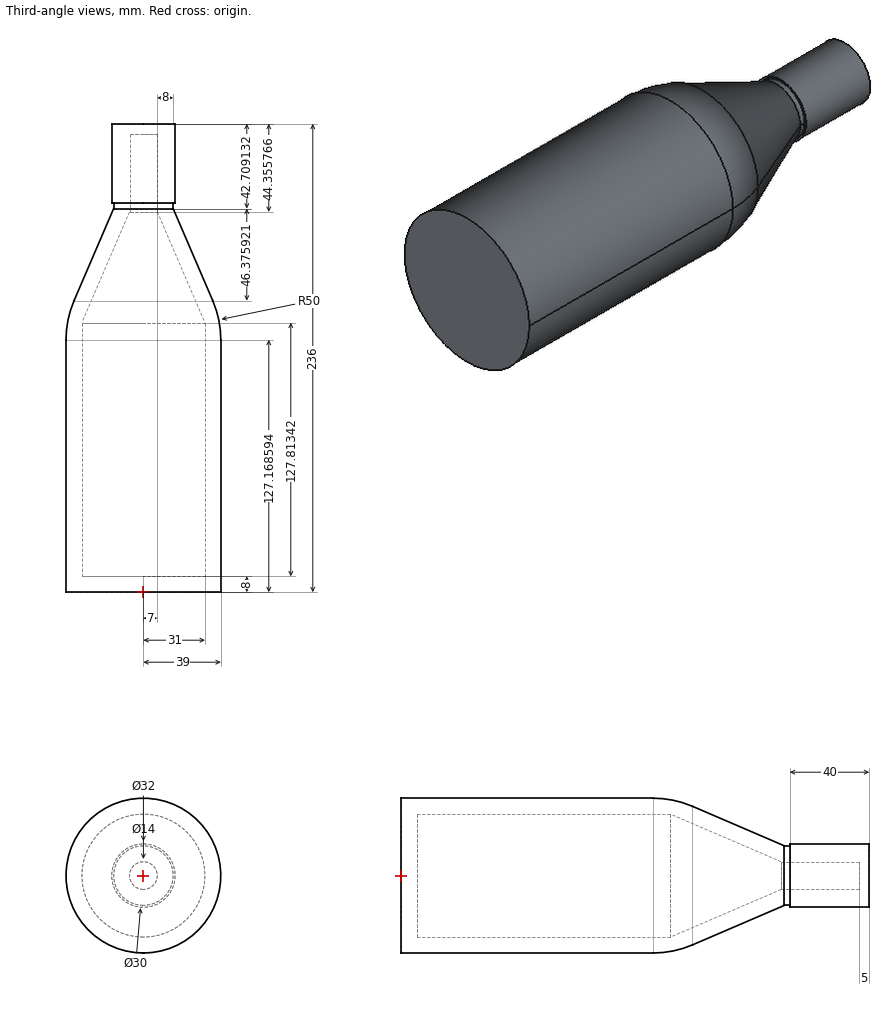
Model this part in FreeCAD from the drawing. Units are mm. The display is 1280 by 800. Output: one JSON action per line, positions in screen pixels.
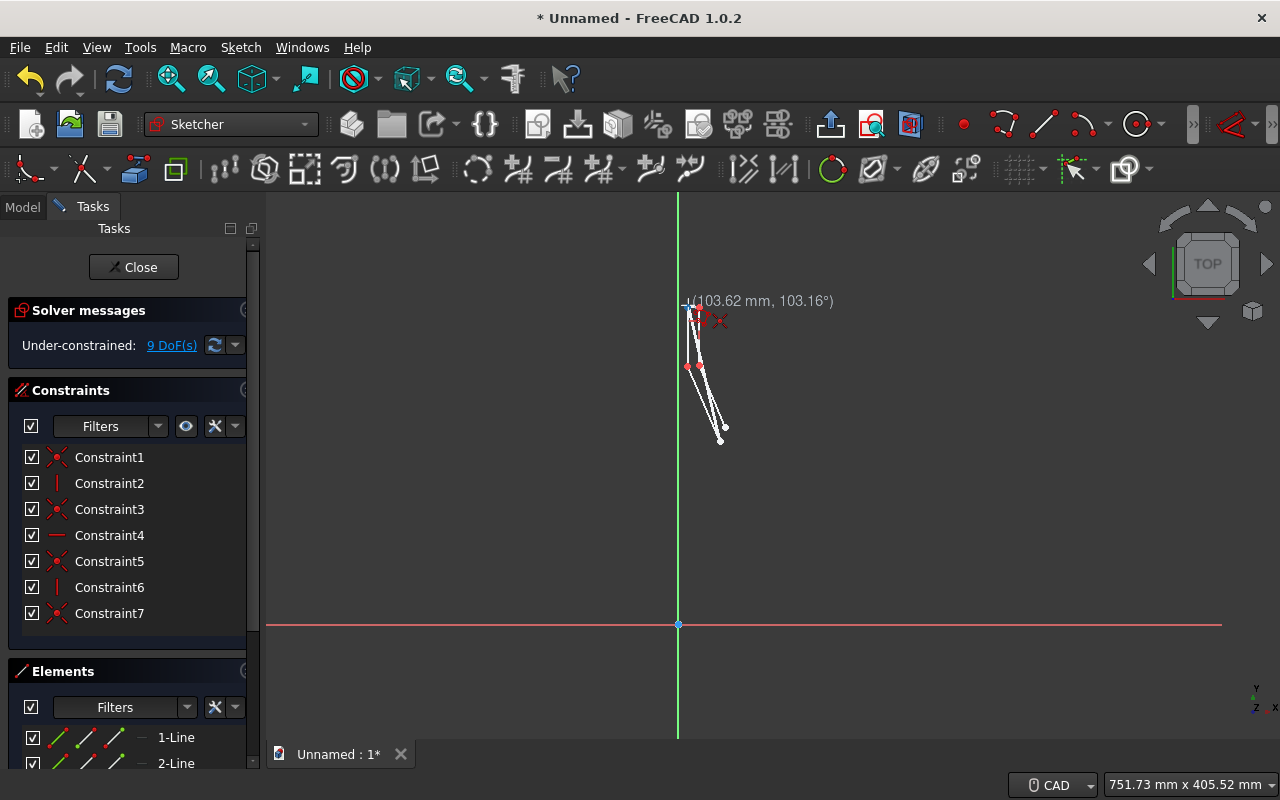
{"action": "scroll", "coordinate": [720, 614], "scroll_direction": "up", "scroll_amount": 2}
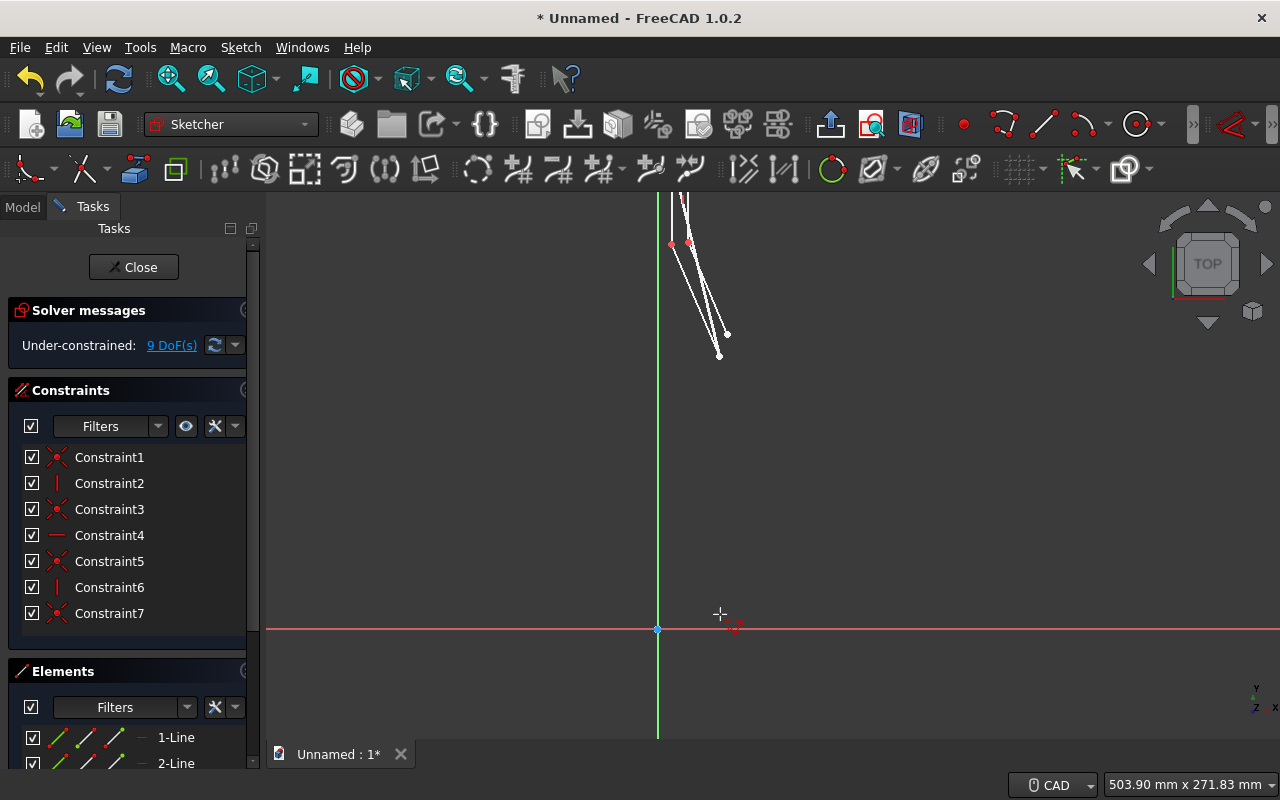
{"action": "left_click", "coordinate": [720, 613]}
{"action": "left_click", "coordinate": [658, 613]}
{"action": "left_click", "coordinate": [658, 629]}
{"action": "left_click", "coordinate": [736, 620]}
{"action": "left_click", "coordinate": [736, 374]}
{"action": "right_click", "coordinate": [736, 374]}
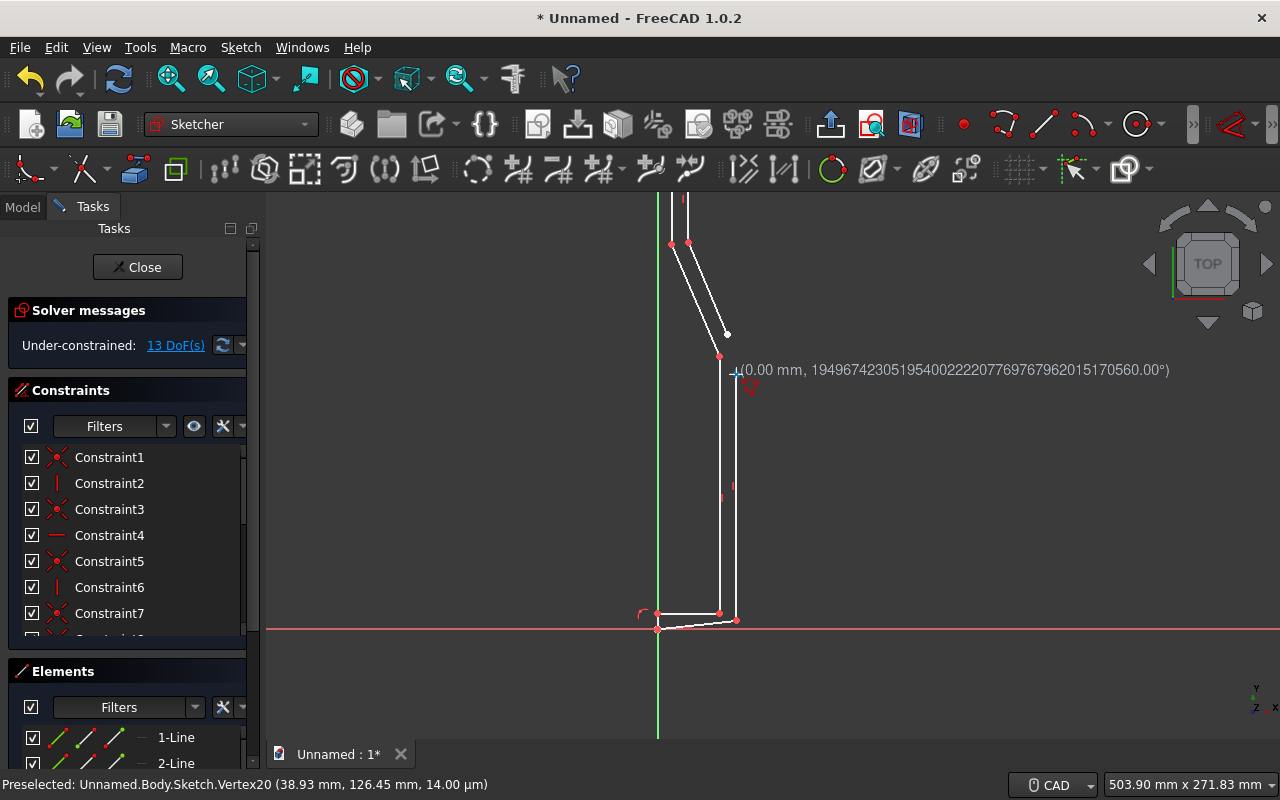
{"action": "key", "text": "g 3 a"}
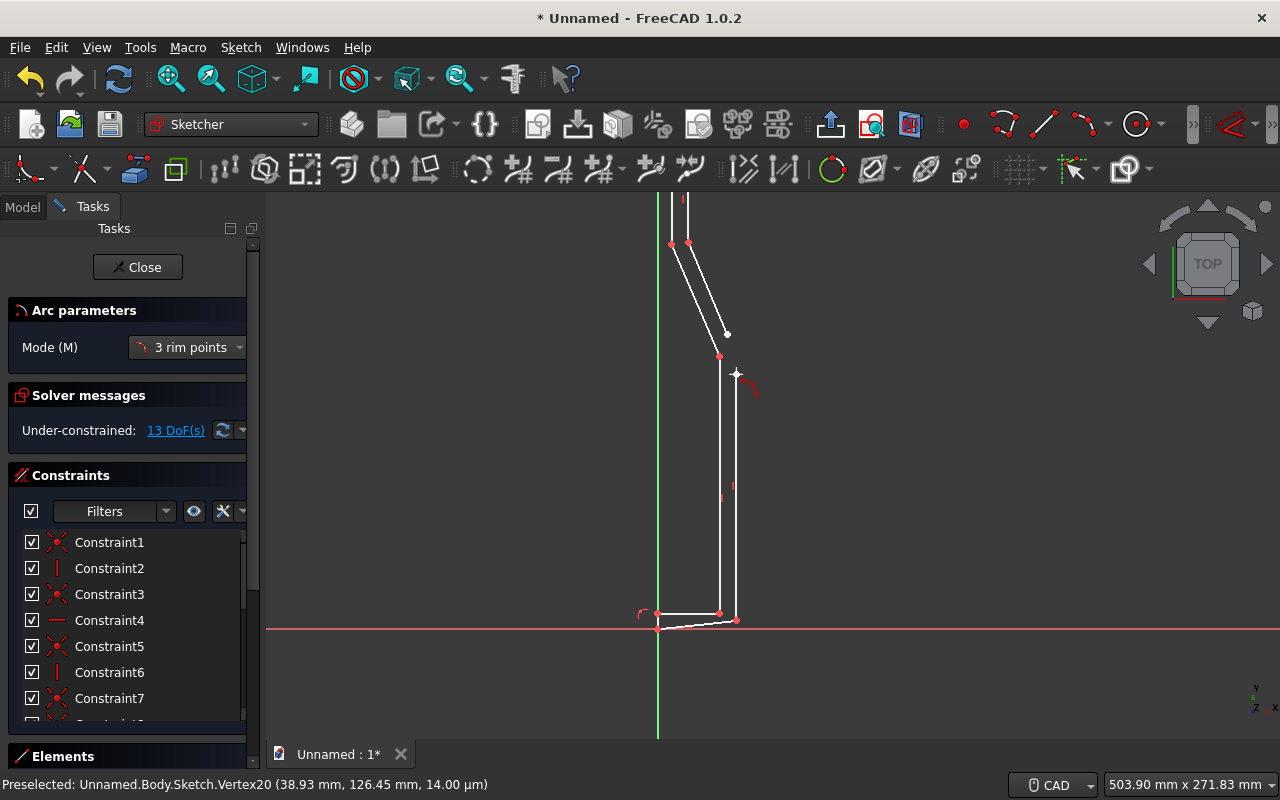
{"action": "left_click", "coordinate": [736, 375]}
{"action": "left_click", "coordinate": [727, 335]}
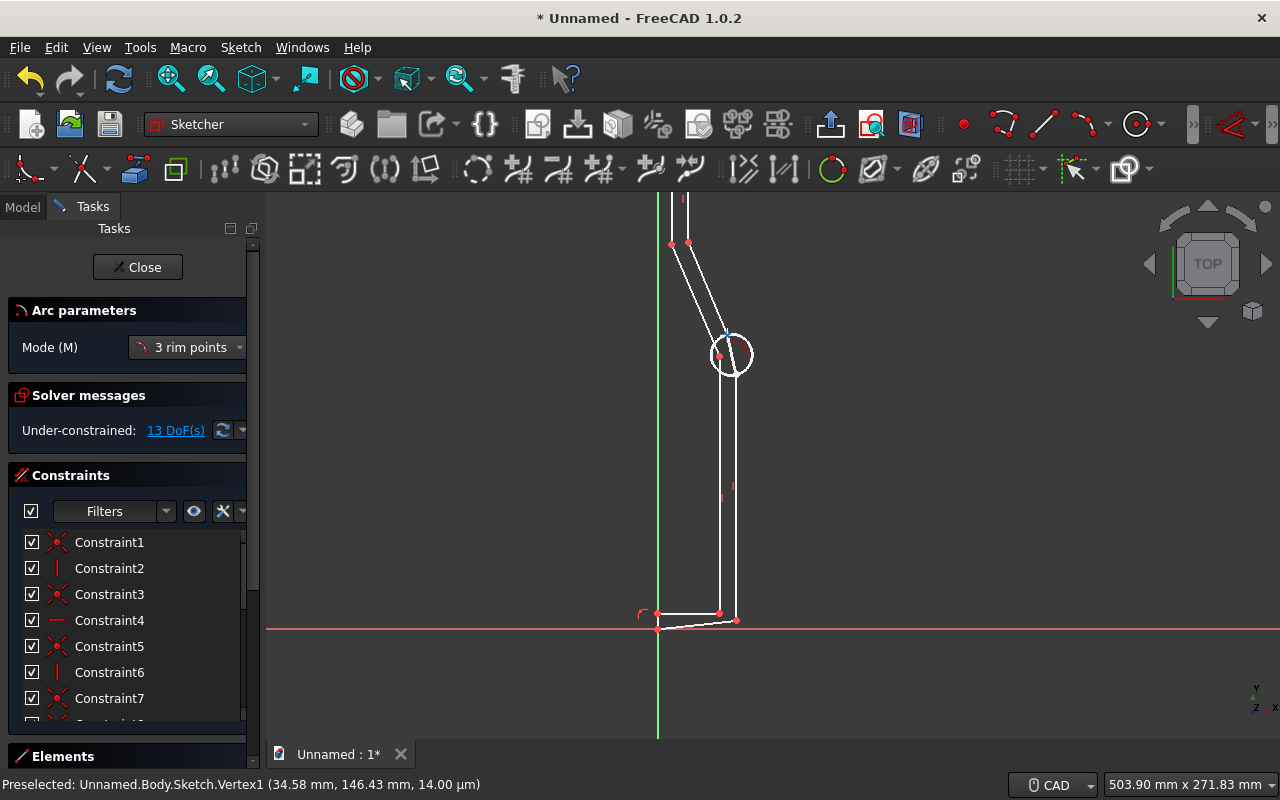
{"action": "scroll", "coordinate": [734, 353], "scroll_direction": "up", "scroll_amount": 11}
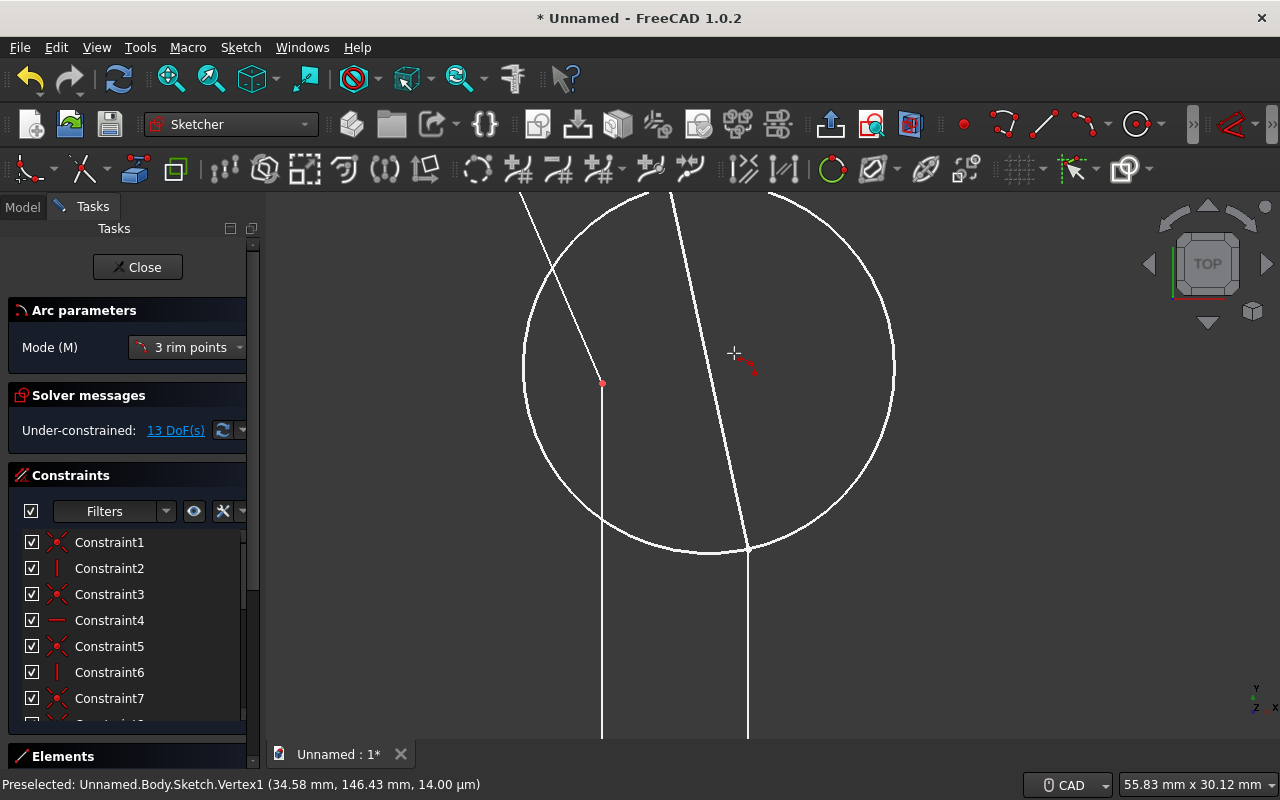
{"action": "left_click", "coordinate": [731, 353]}
{"action": "key", "text": "Escape"}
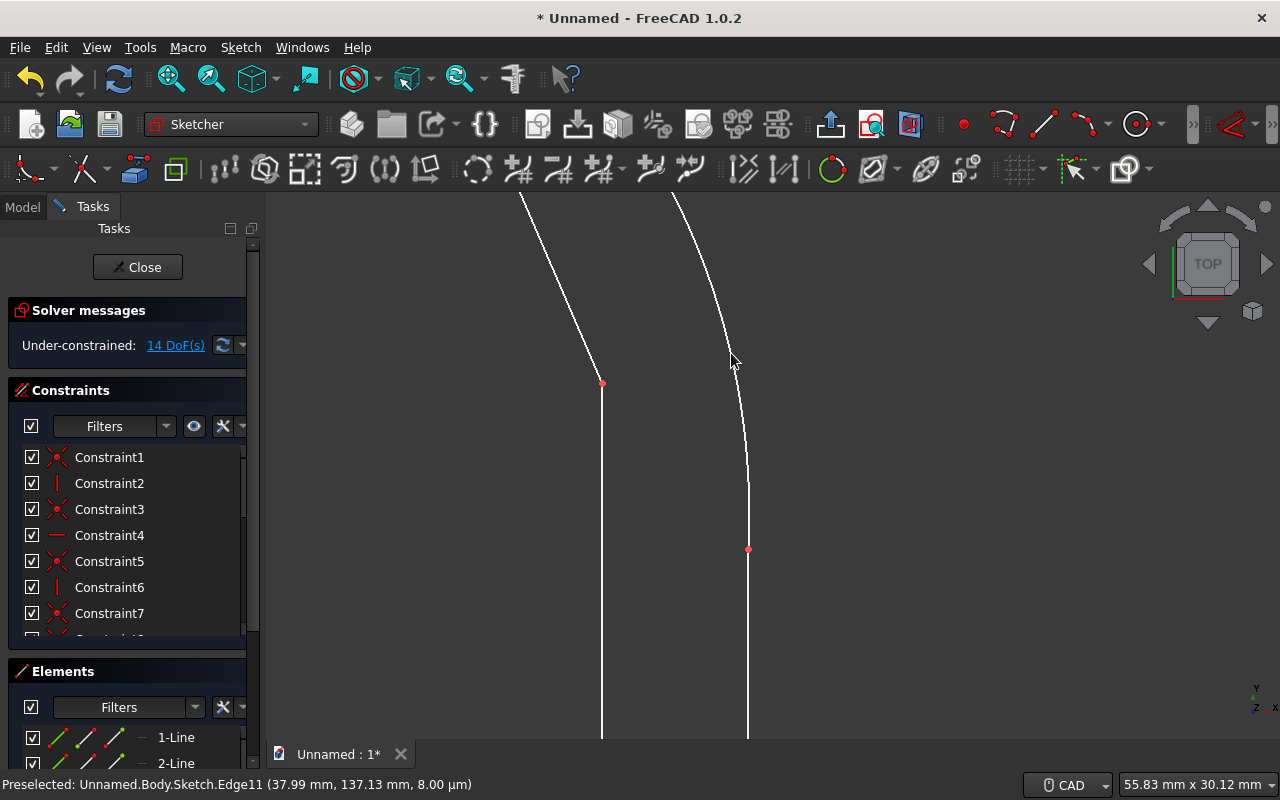
{"action": "scroll", "coordinate": [729, 446], "scroll_direction": "down", "scroll_amount": 13}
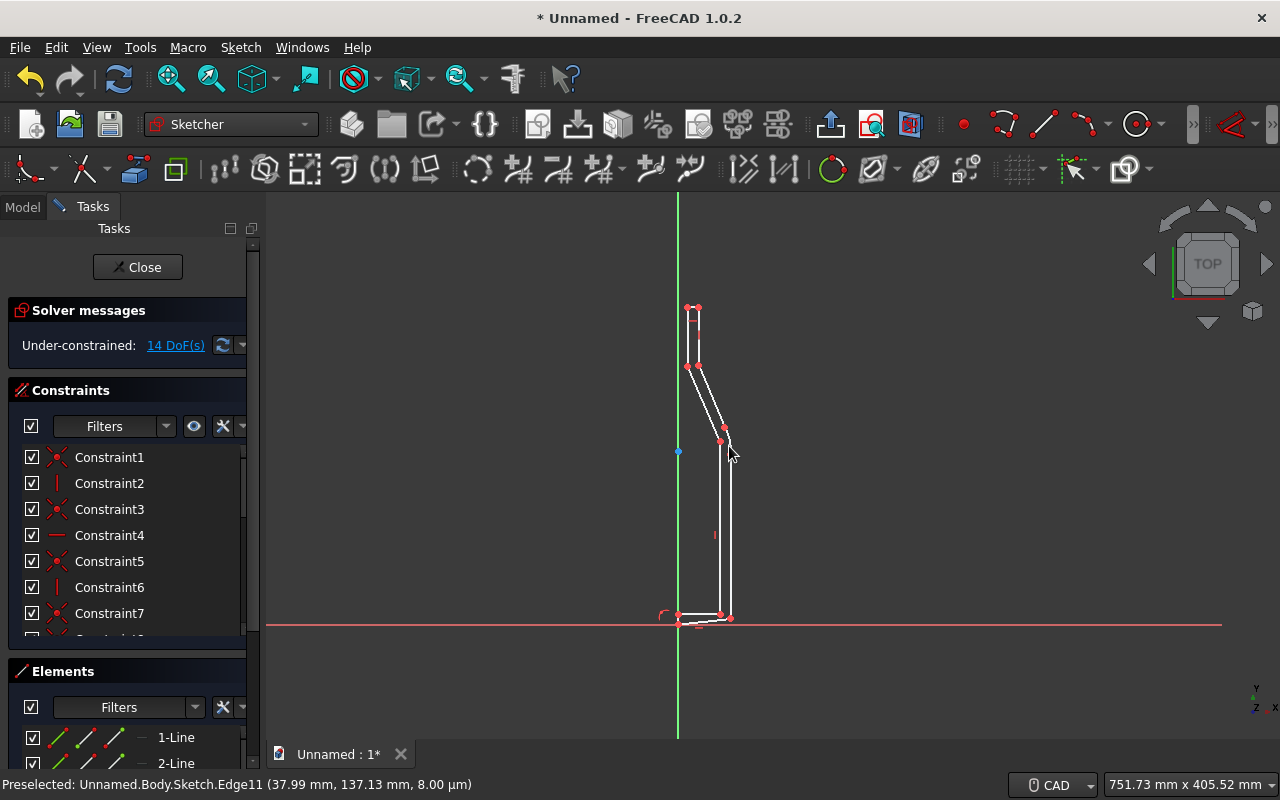
{"action": "scroll", "coordinate": [717, 409], "scroll_direction": "up", "scroll_amount": 2}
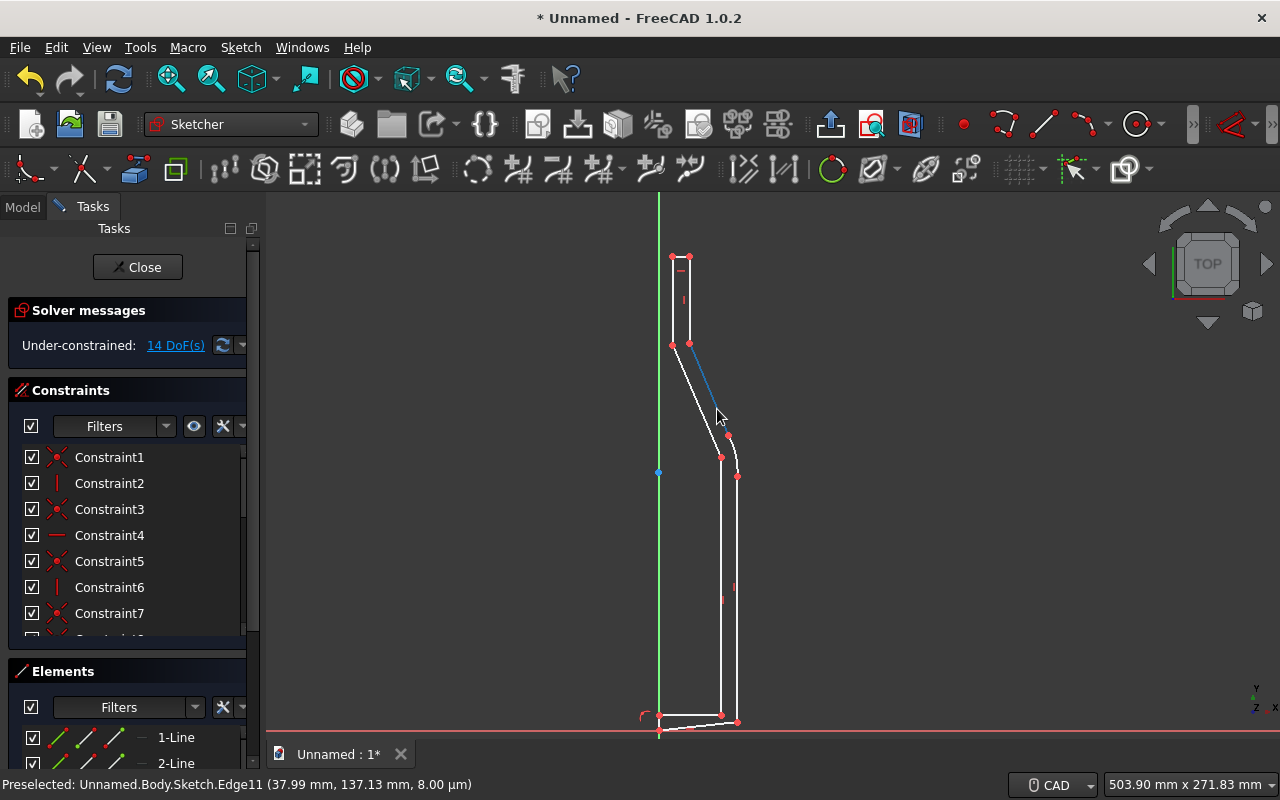
{"action": "left_click", "coordinate": [717, 408]}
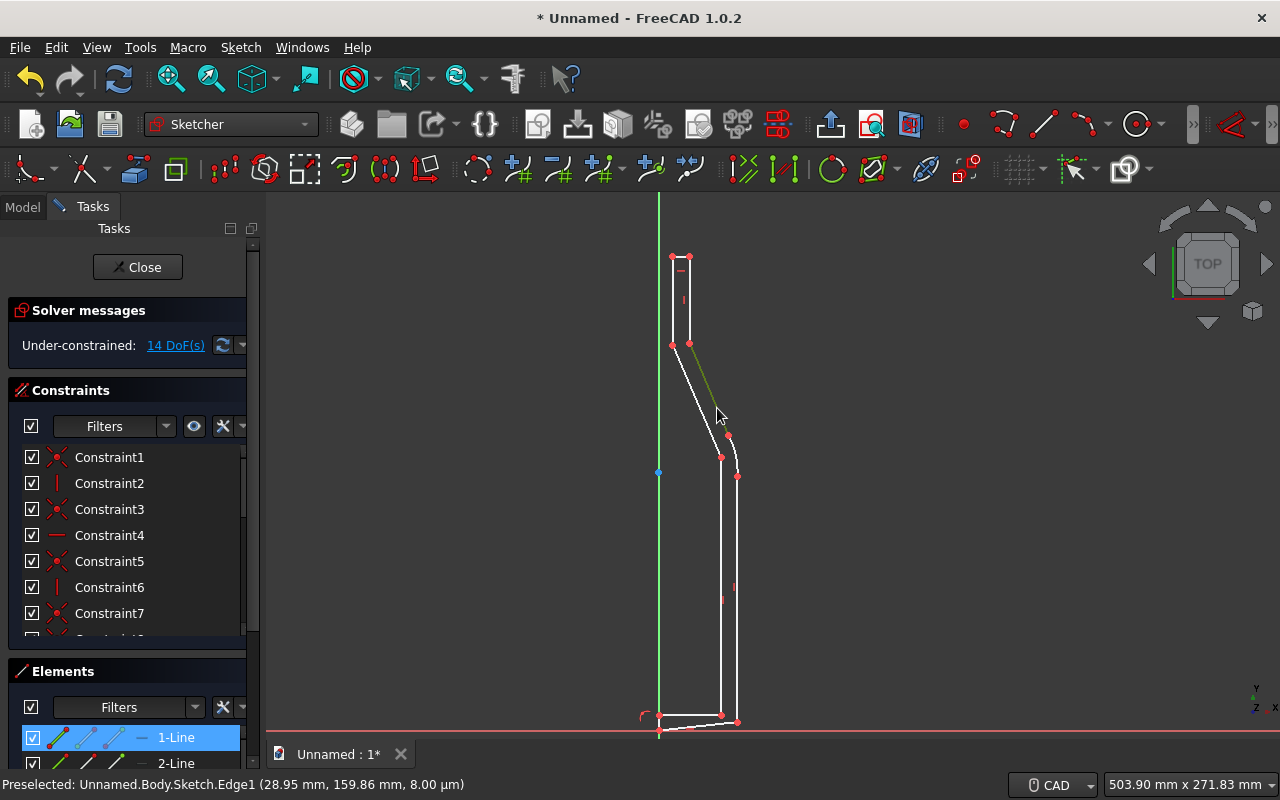
{"action": "left_click", "coordinate": [737, 464]}